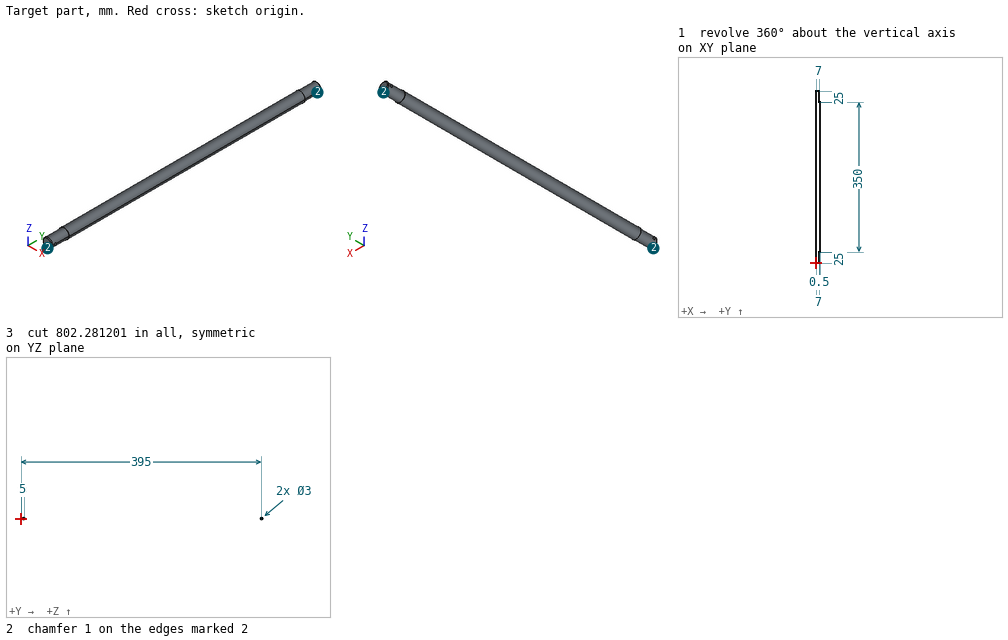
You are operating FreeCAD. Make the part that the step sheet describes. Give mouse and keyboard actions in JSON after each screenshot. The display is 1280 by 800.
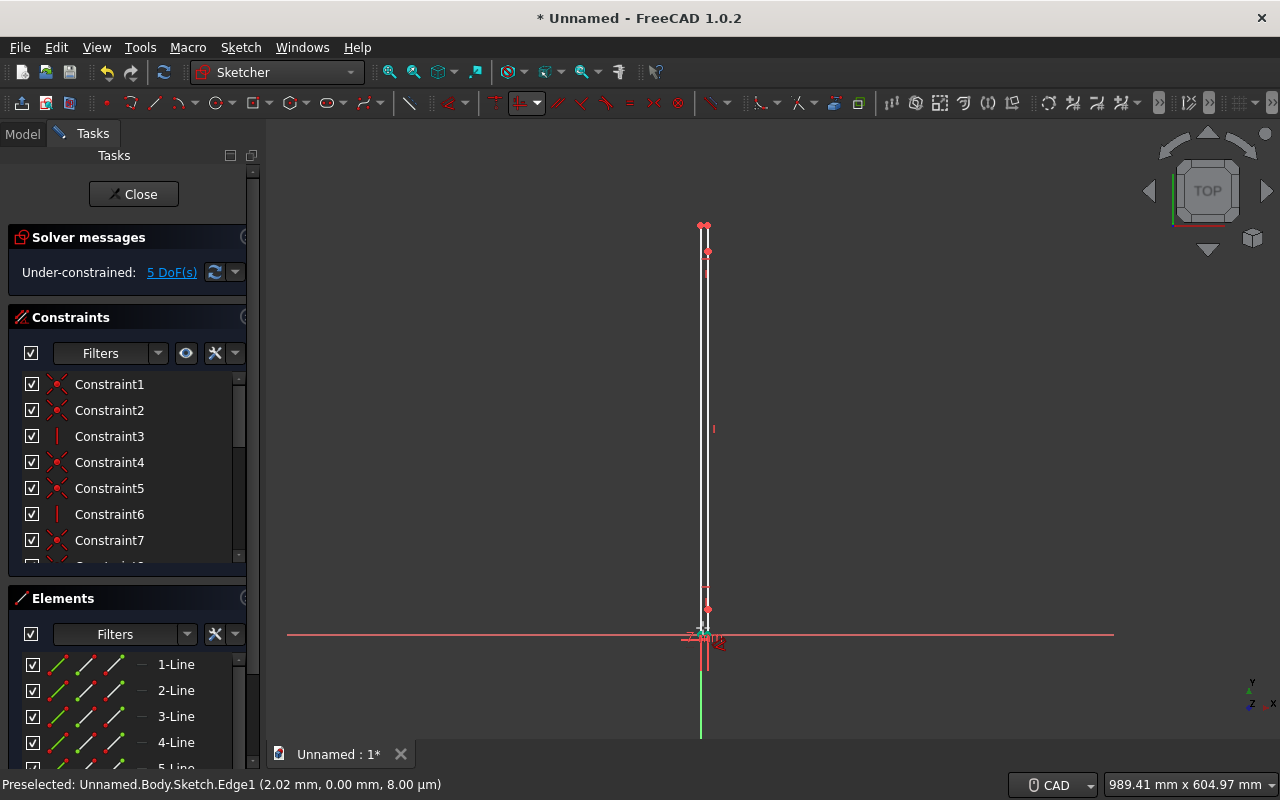
{"action": "scroll", "coordinate": [706, 225], "scroll_direction": "up", "scroll_amount": 10}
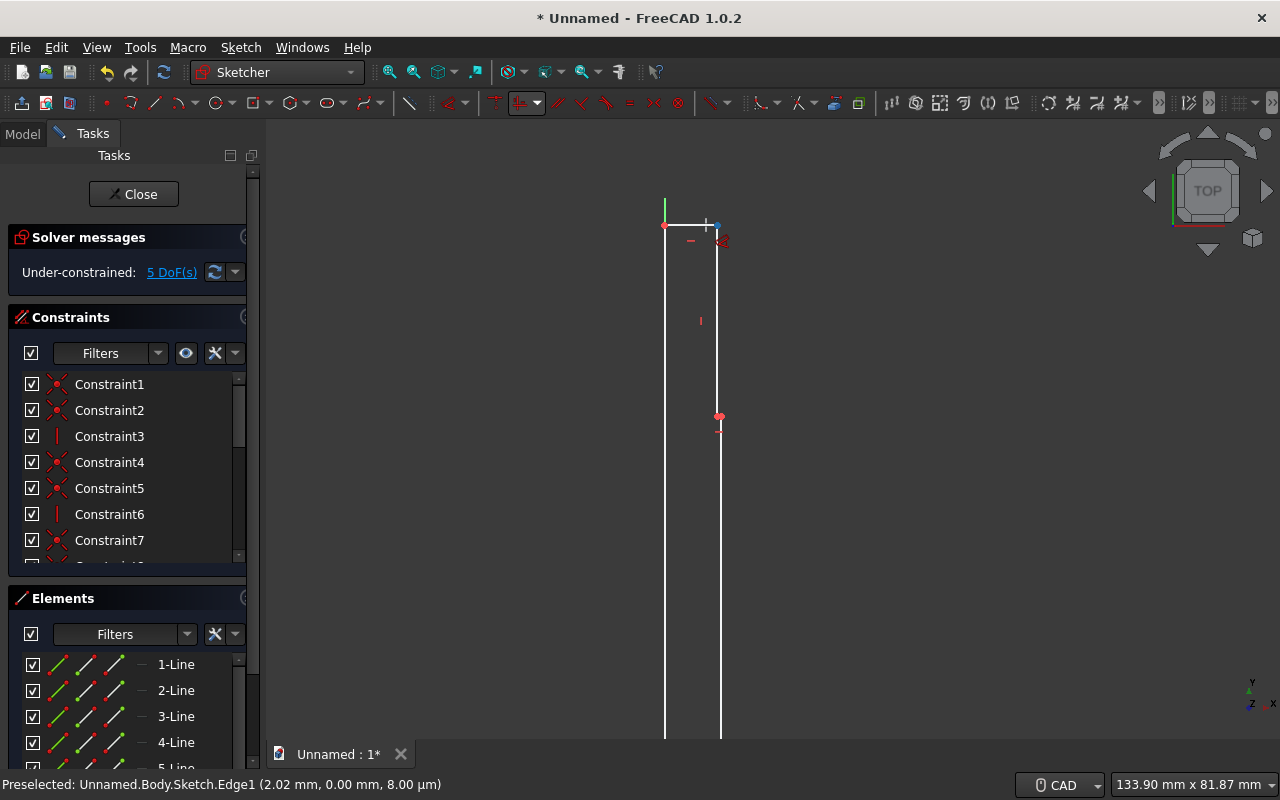
{"action": "left_click", "coordinate": [702, 225]}
{"action": "left_click", "coordinate": [691, 191]}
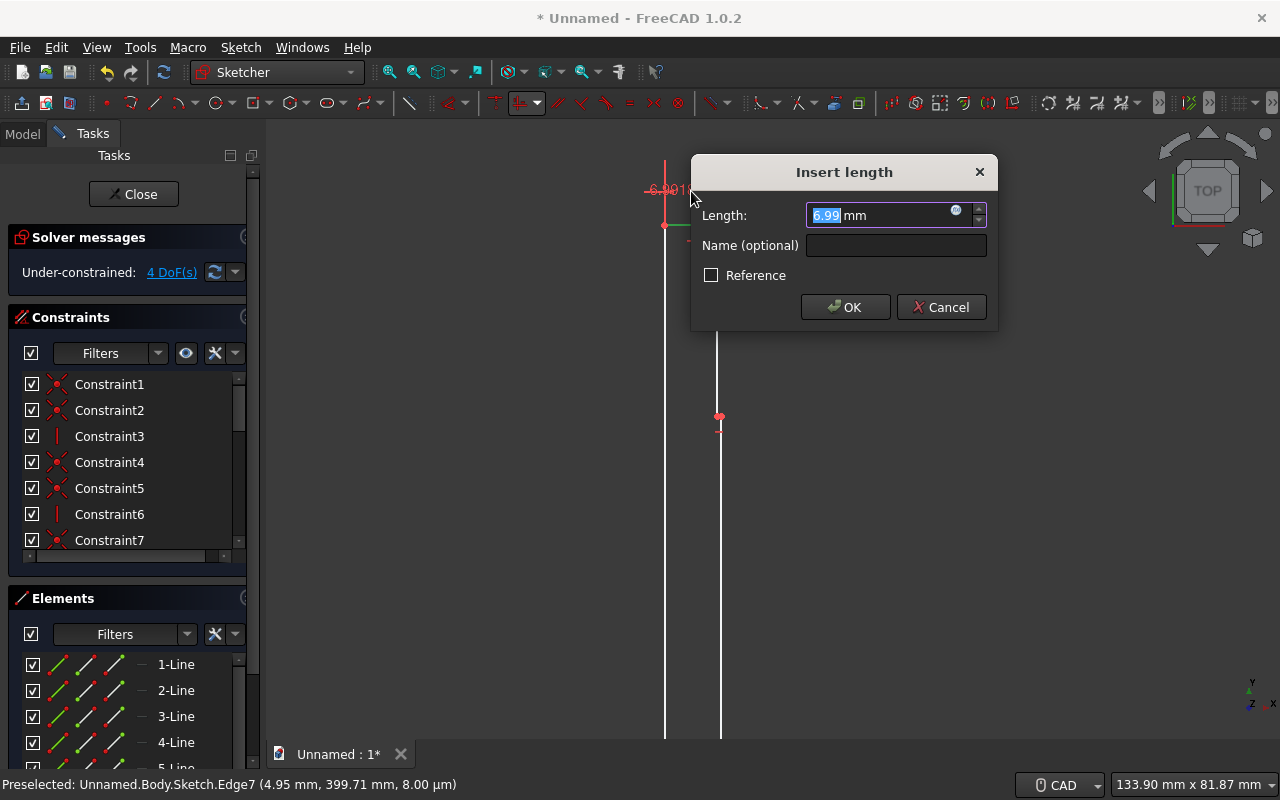
{"action": "type", "text": "7"}
{"action": "key", "text": "Return"}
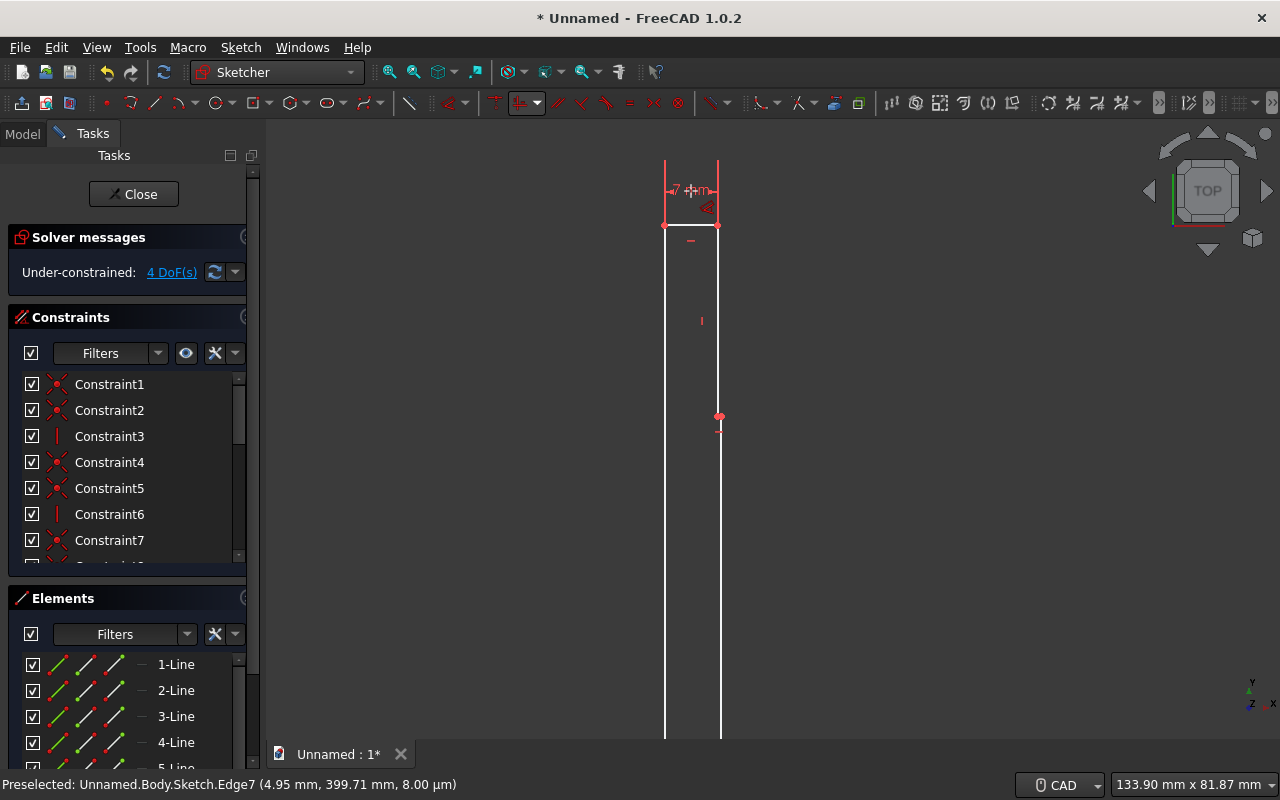
{"action": "scroll", "coordinate": [706, 224], "scroll_direction": "down", "scroll_amount": 10}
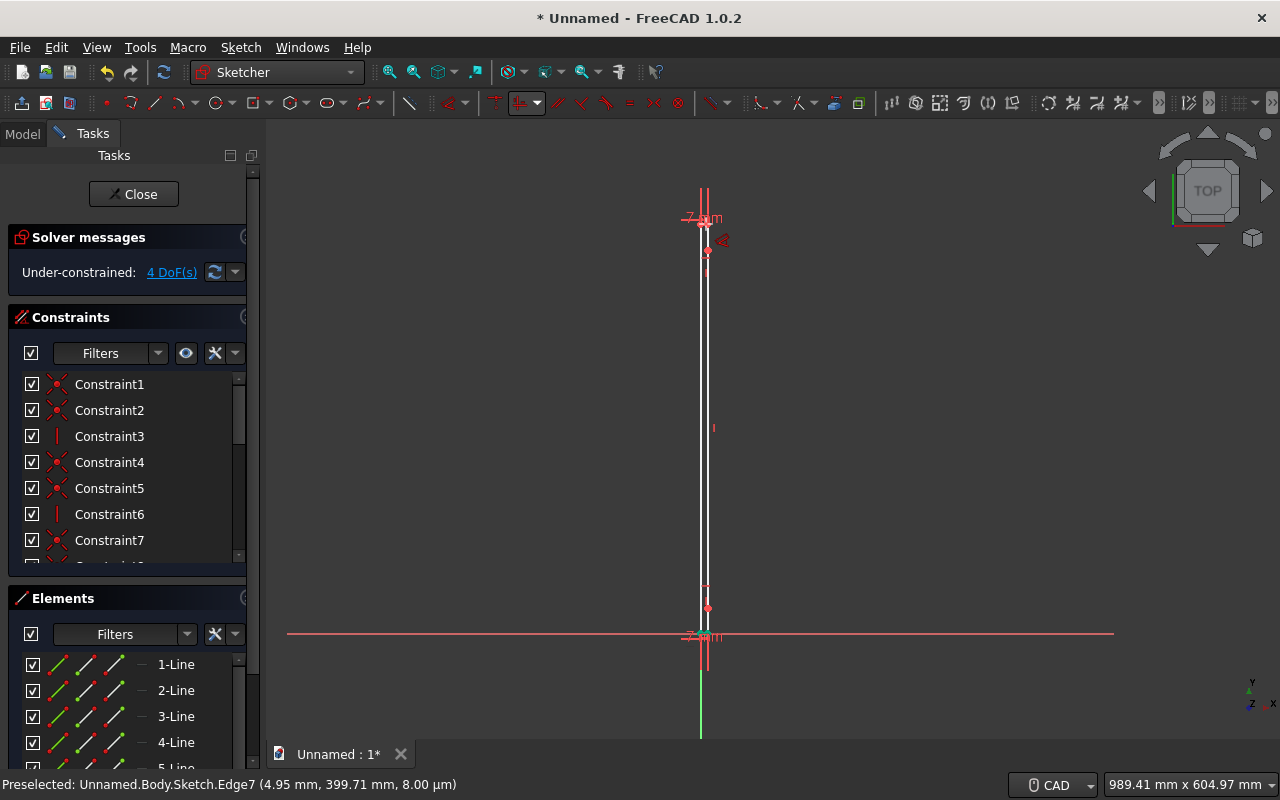
{"action": "scroll", "coordinate": [708, 626], "scroll_direction": "up", "scroll_amount": 4}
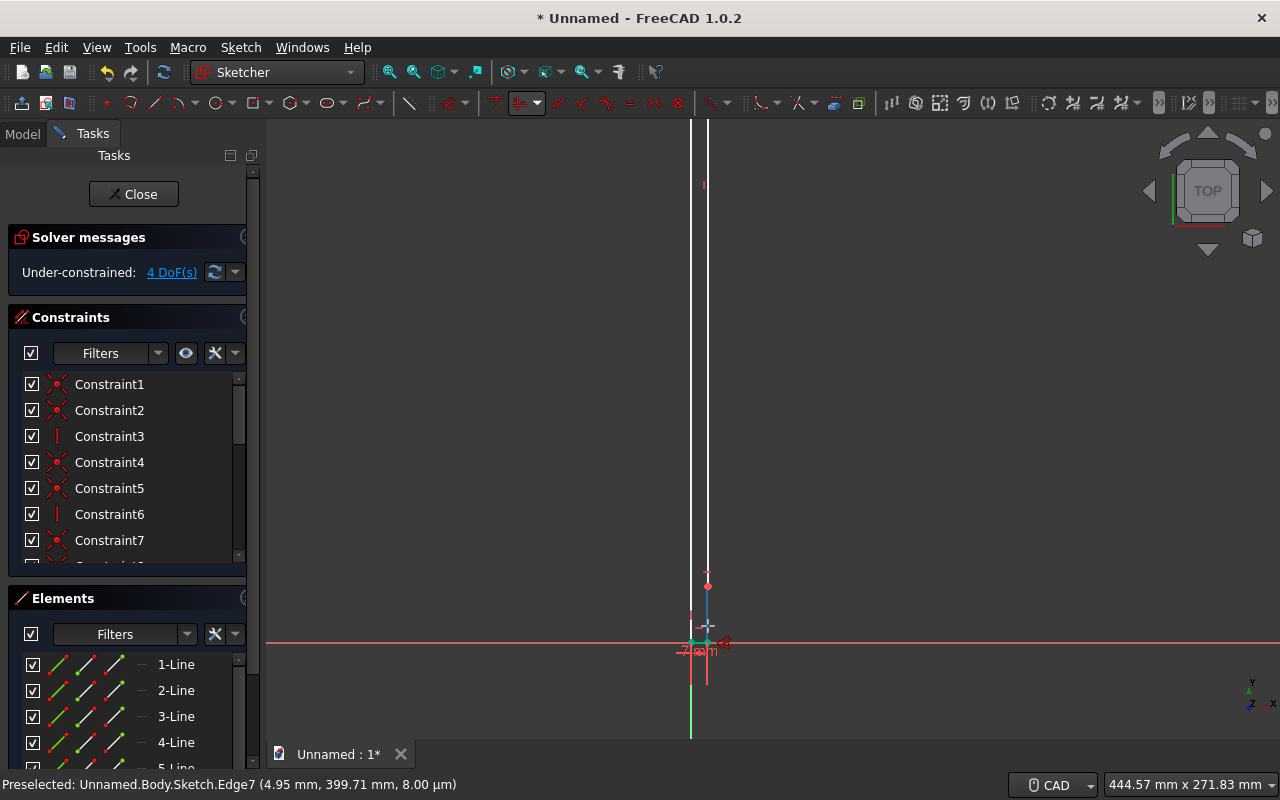
{"action": "left_click", "coordinate": [707, 626]}
{"action": "left_click", "coordinate": [741, 615]}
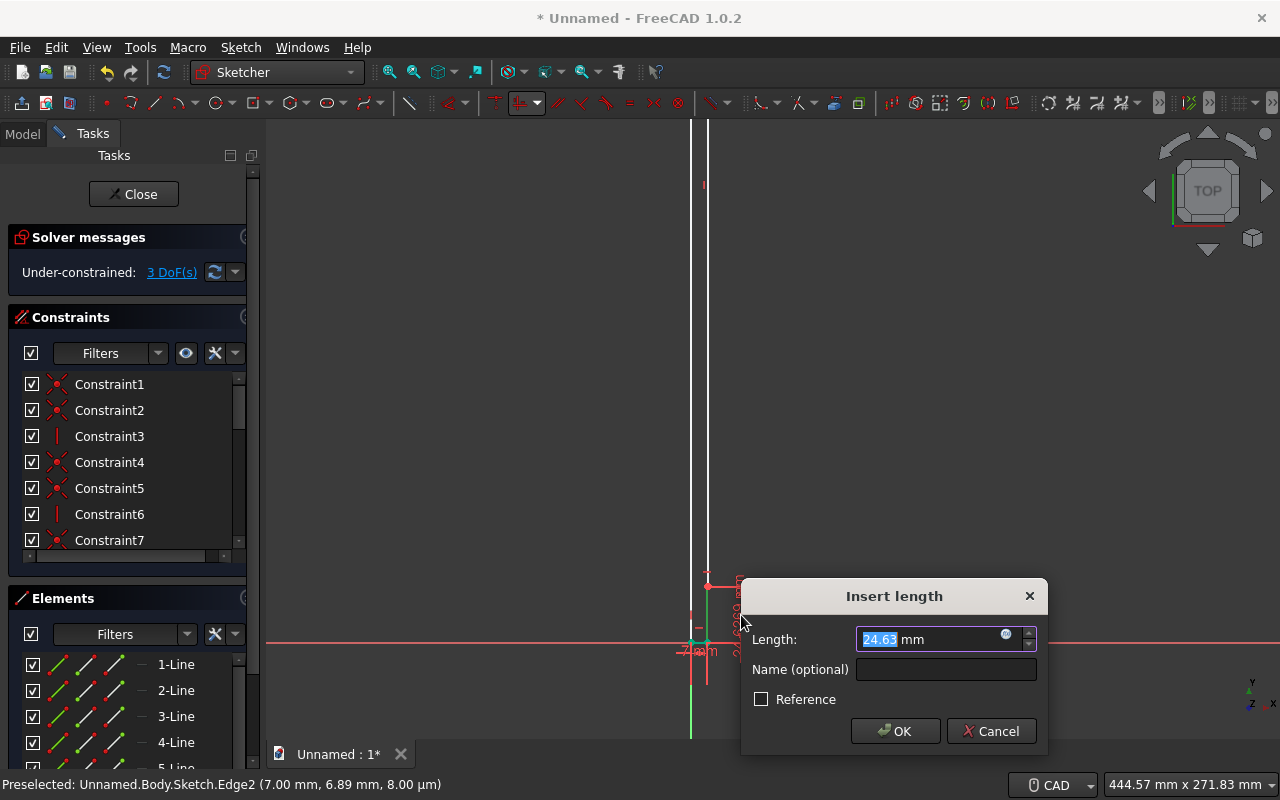
{"action": "type", "text": "25"}
{"action": "key", "text": "Return"}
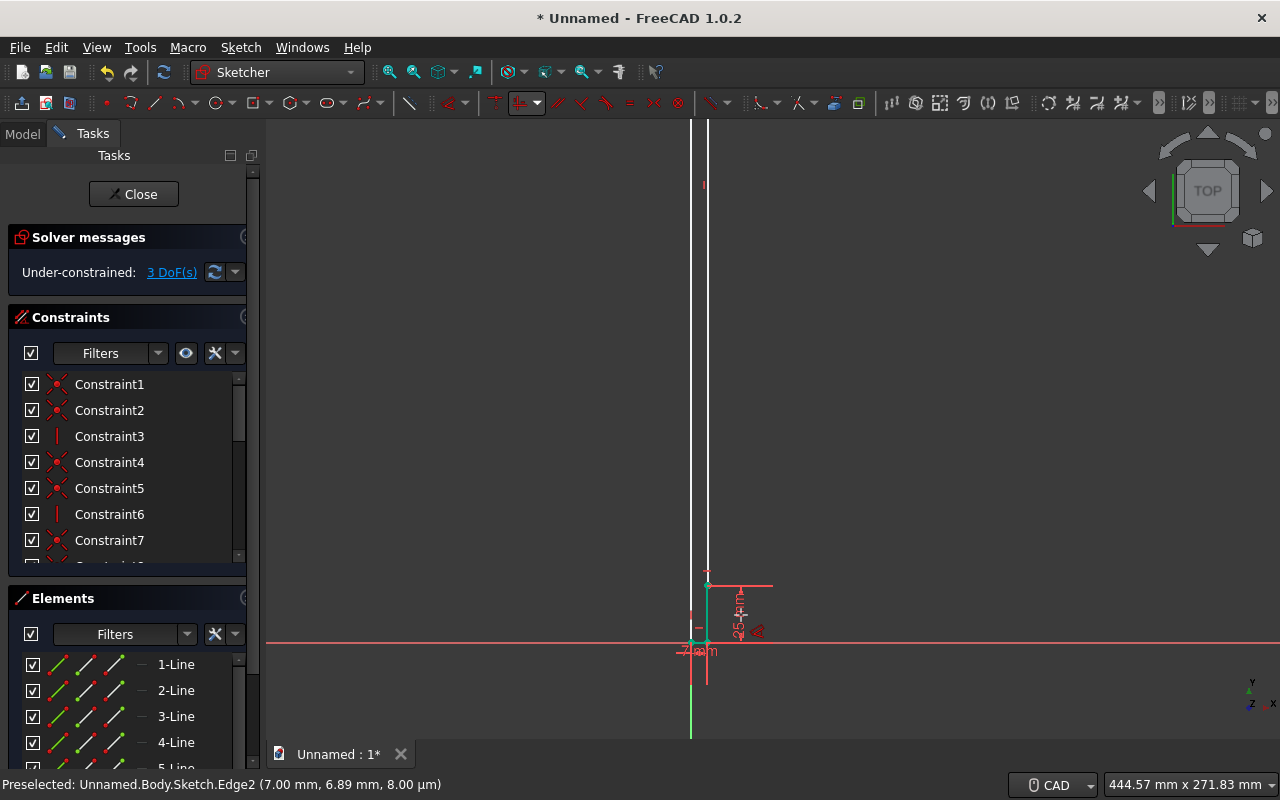
{"action": "scroll", "coordinate": [708, 627], "scroll_direction": "down", "scroll_amount": 4}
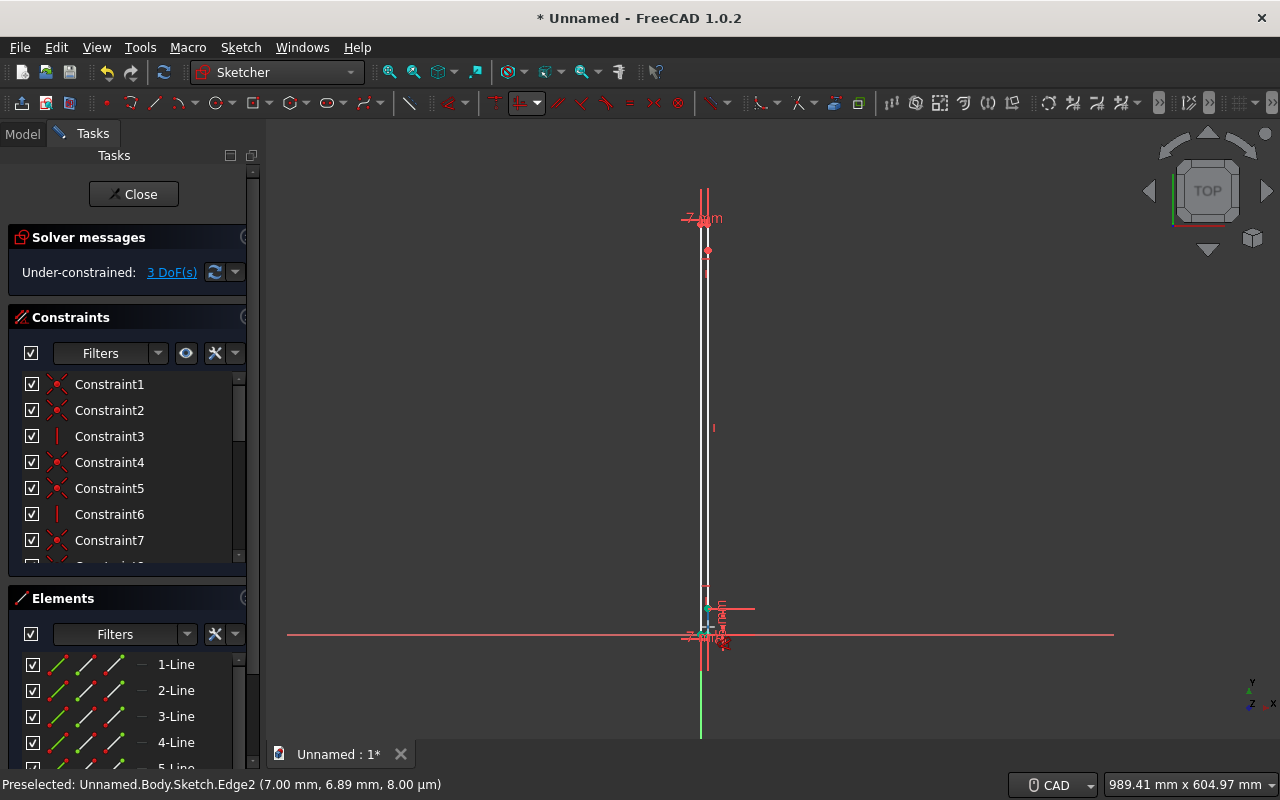
{"action": "scroll", "coordinate": [708, 243], "scroll_direction": "up", "scroll_amount": 4}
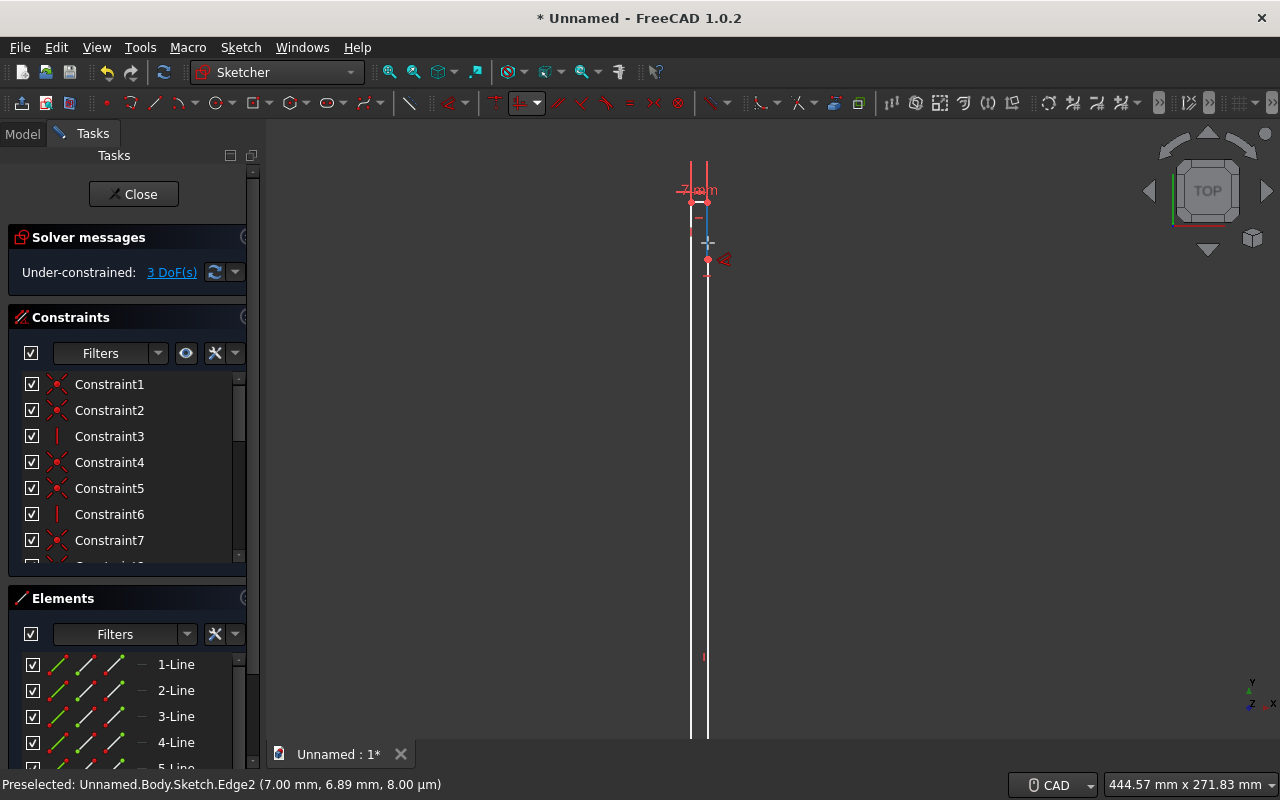
{"action": "left_click", "coordinate": [707, 243]}
{"action": "left_click", "coordinate": [741, 231]}